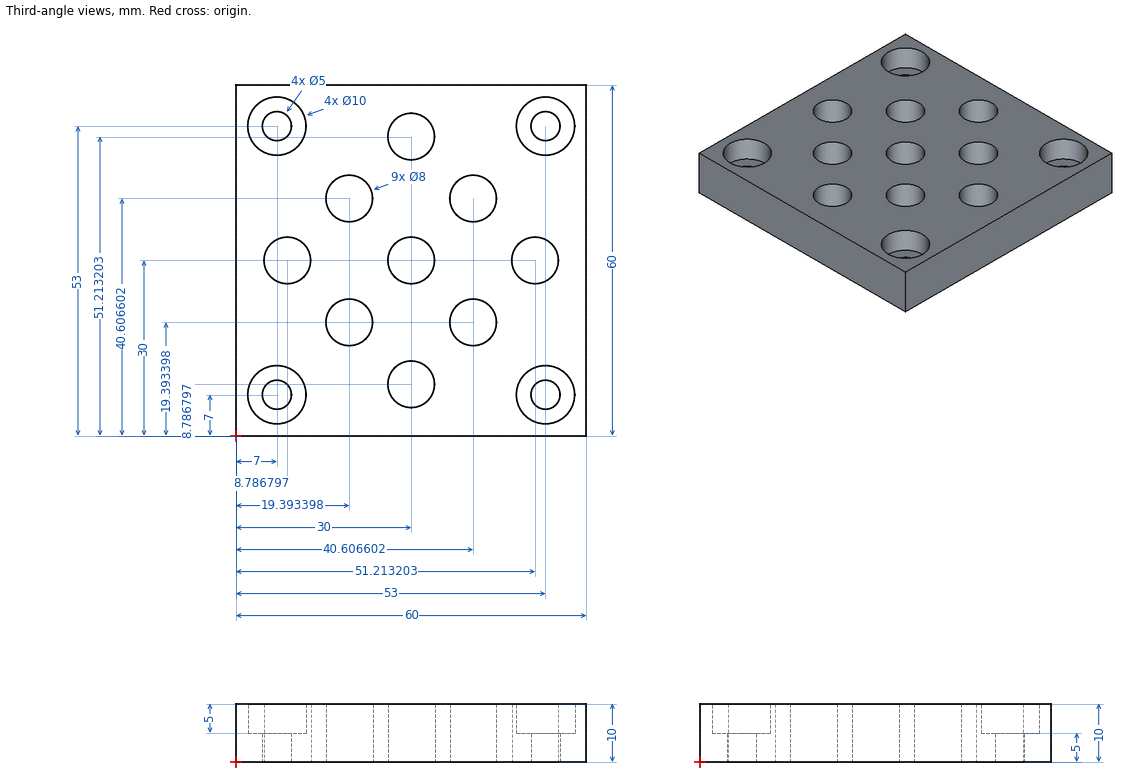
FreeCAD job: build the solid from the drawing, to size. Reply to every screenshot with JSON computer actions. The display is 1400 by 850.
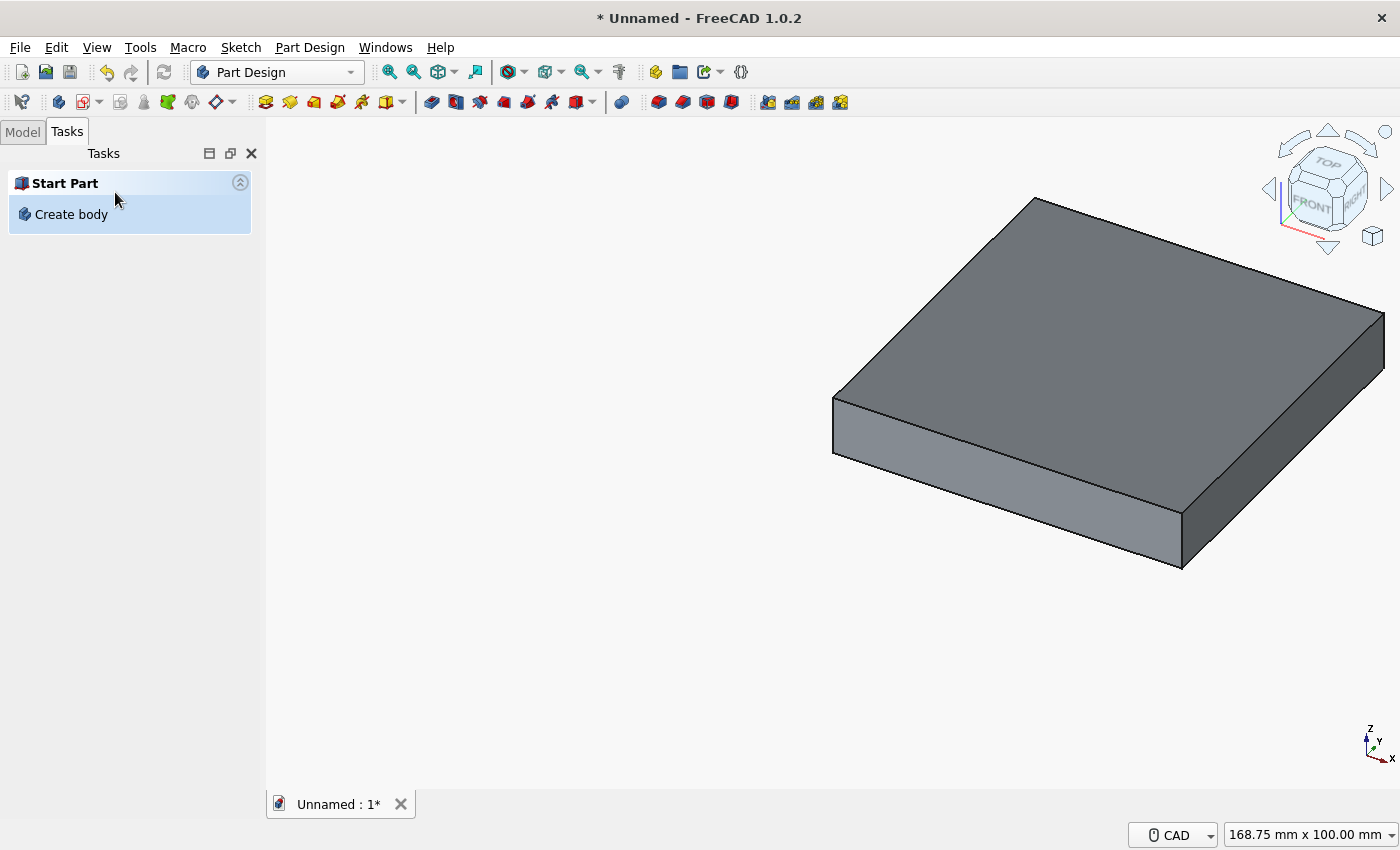
{"action": "left_click", "coordinate": [1108, 355]}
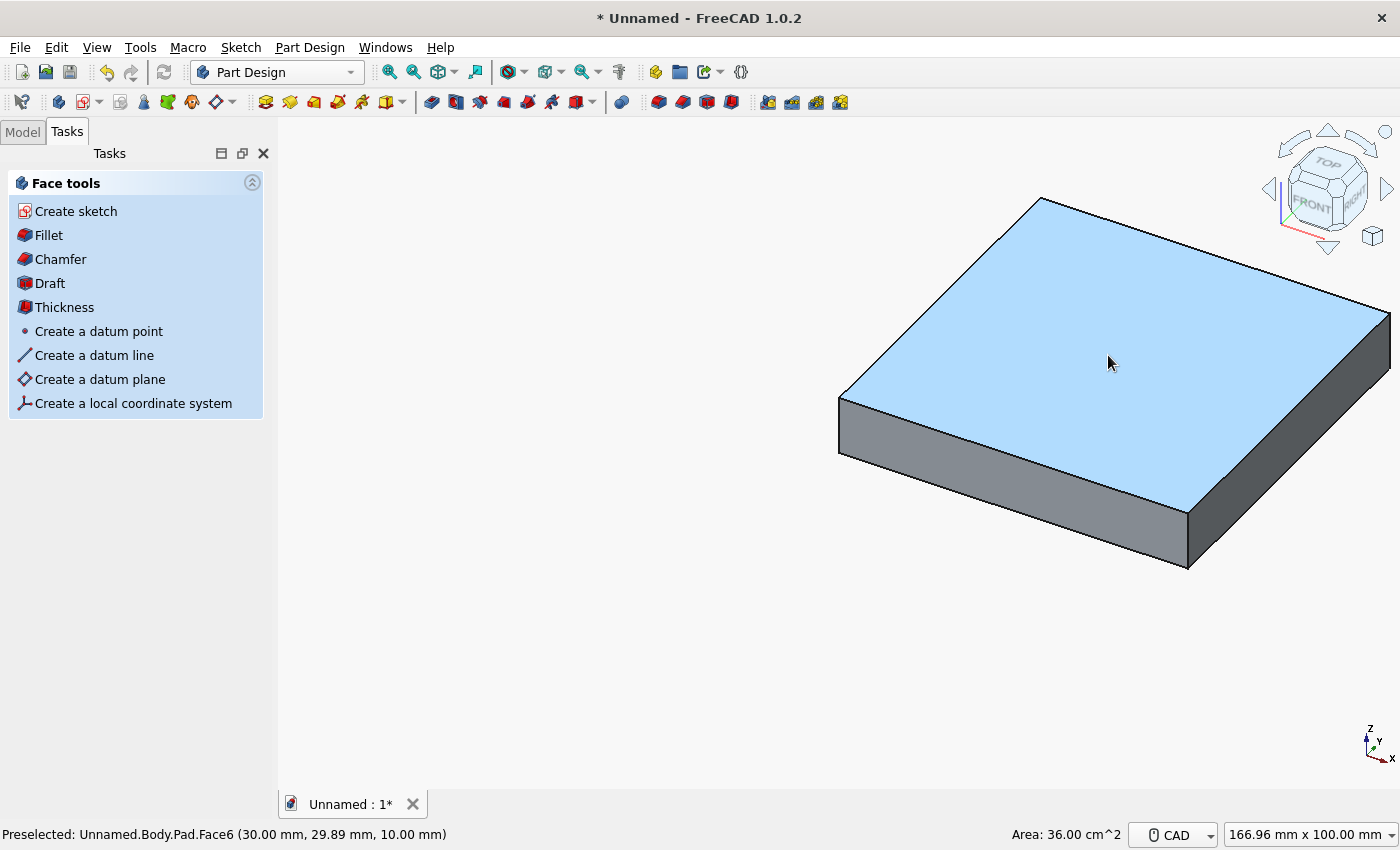
{"action": "left_click", "coordinate": [84, 102]}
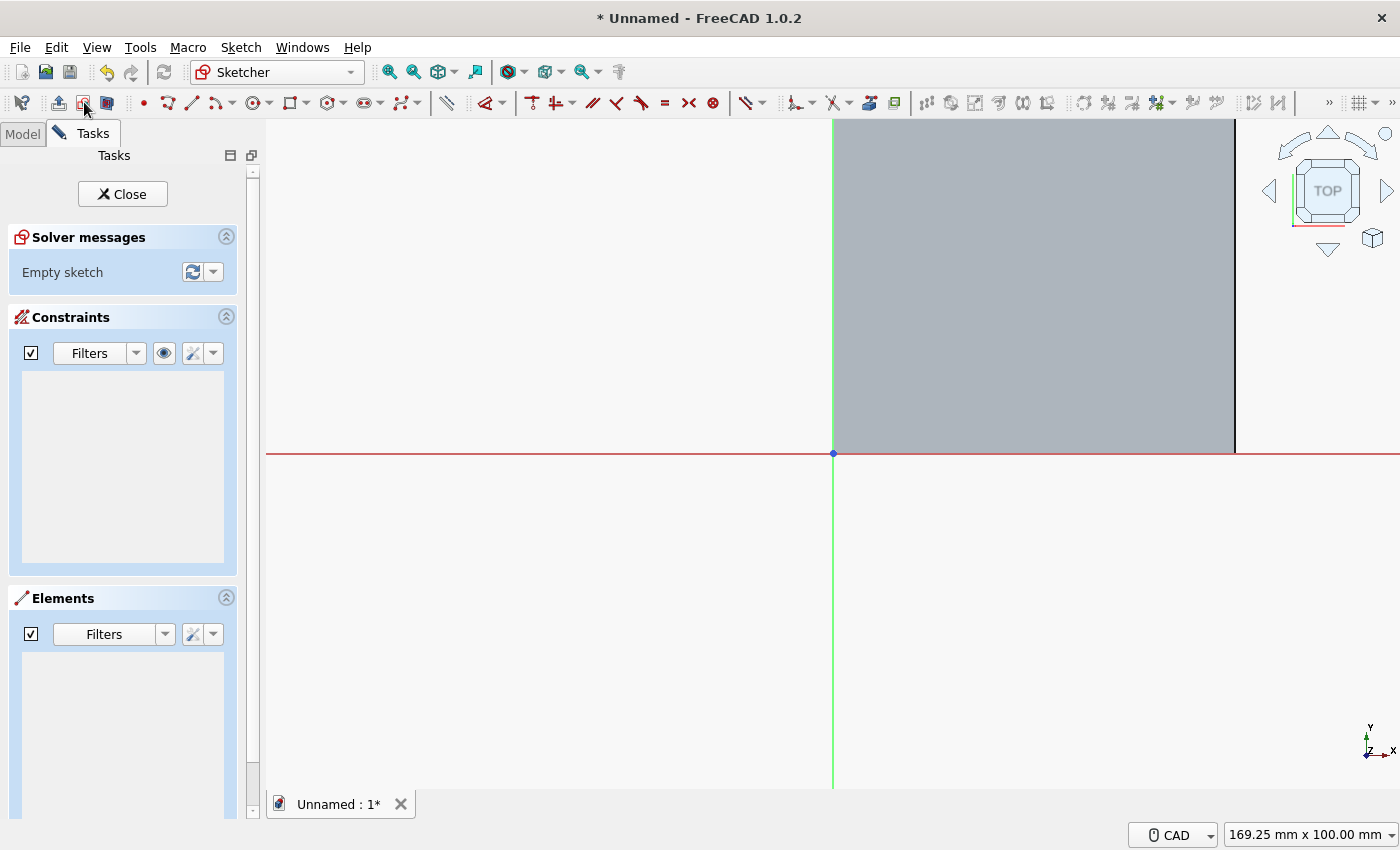
{"action": "scroll", "coordinate": [294, 761], "scroll_direction": "down", "scroll_amount": 1}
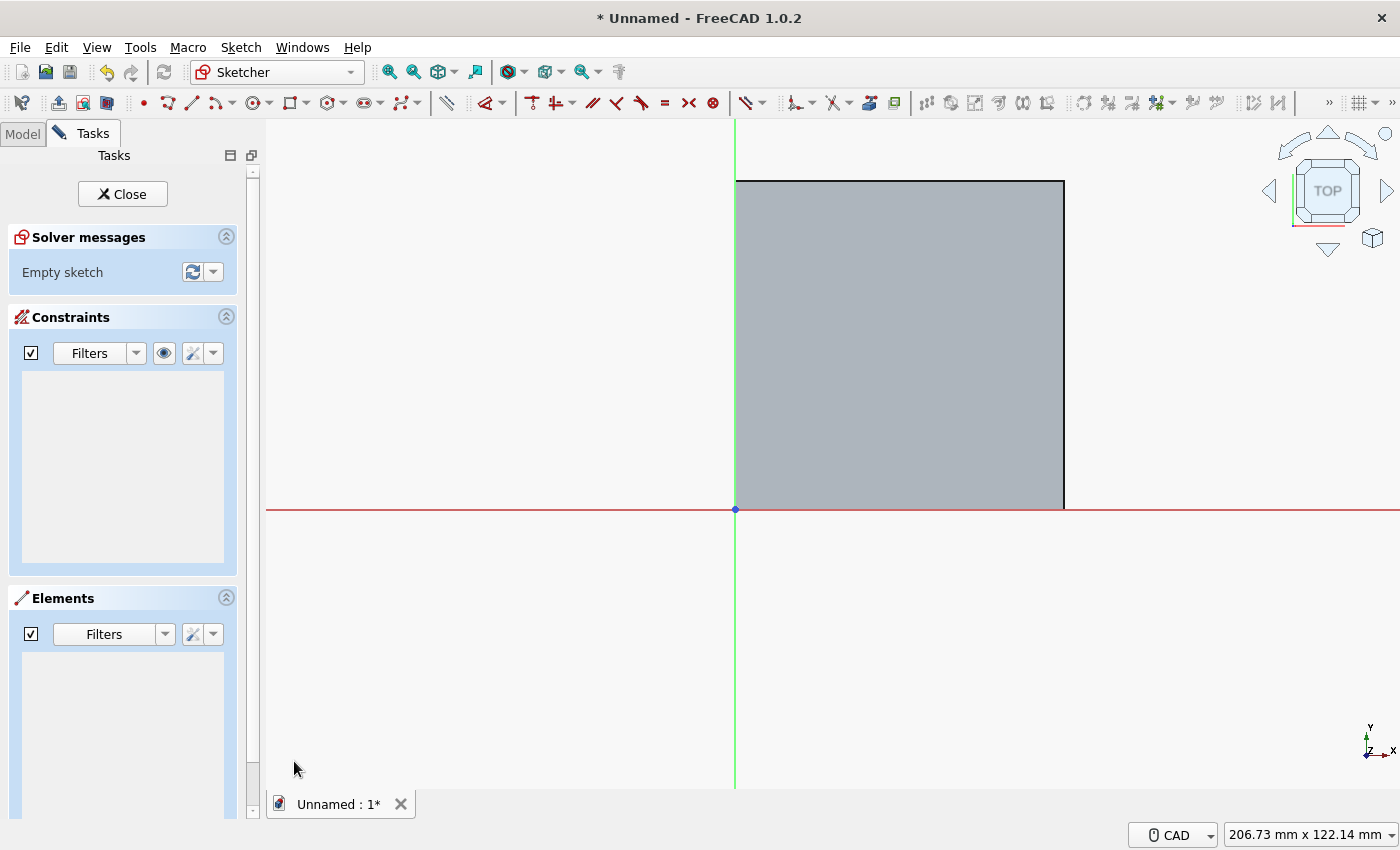
{"action": "scroll", "coordinate": [1158, 147], "scroll_direction": "up", "scroll_amount": 2}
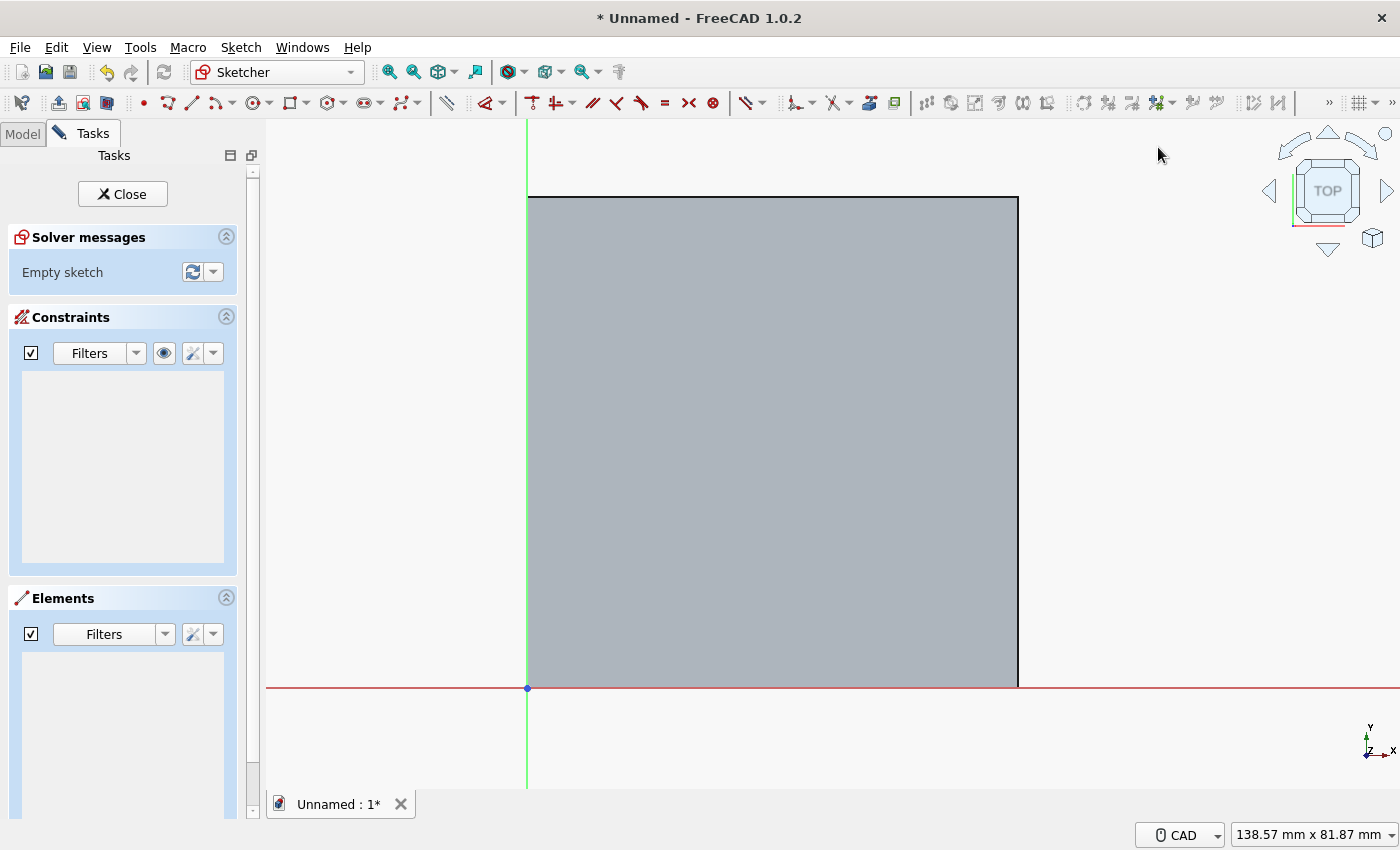
{"action": "left_click", "coordinate": [254, 104]}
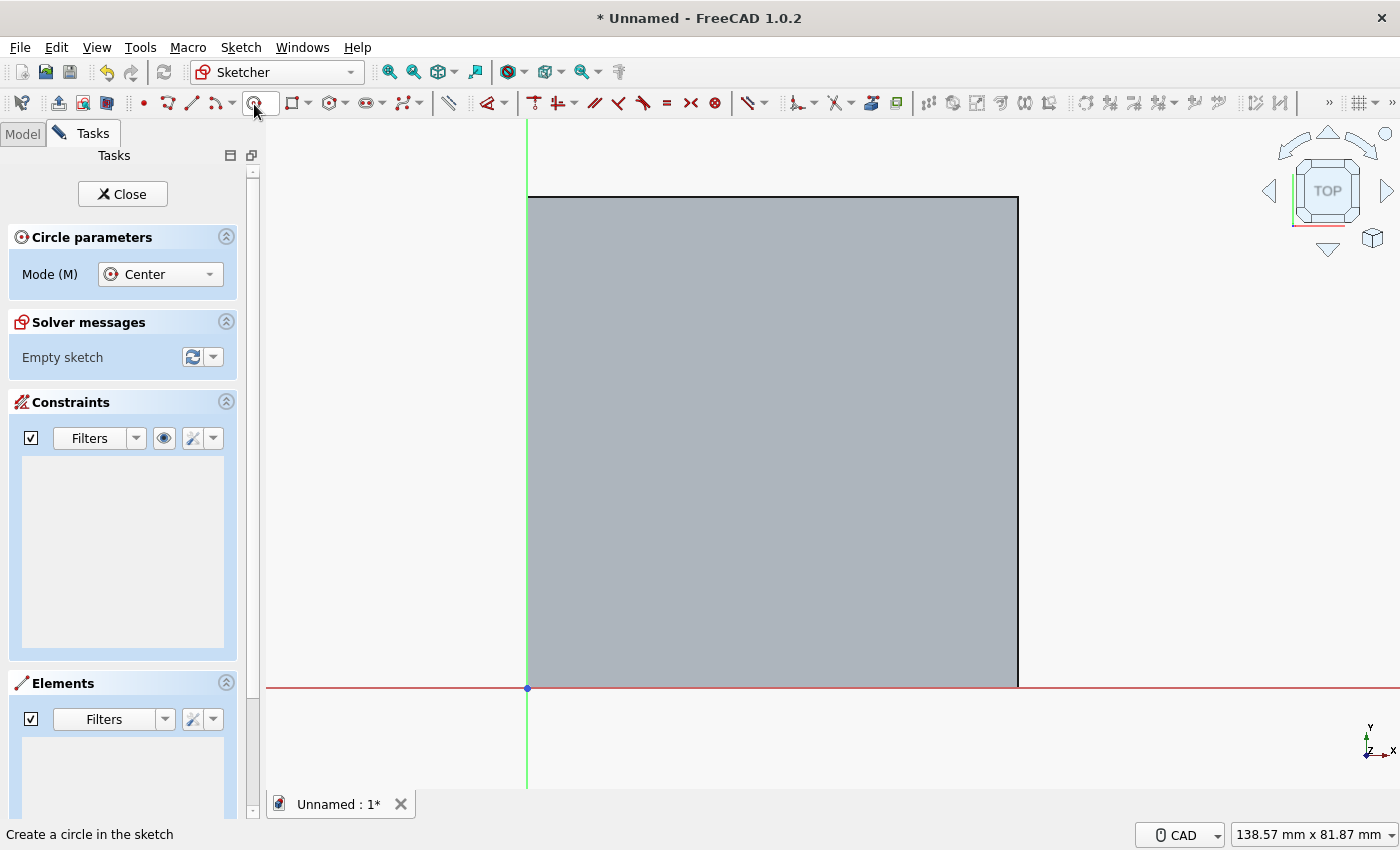
{"action": "left_click", "coordinate": [584, 255]}
{"action": "left_click", "coordinate": [613, 226]}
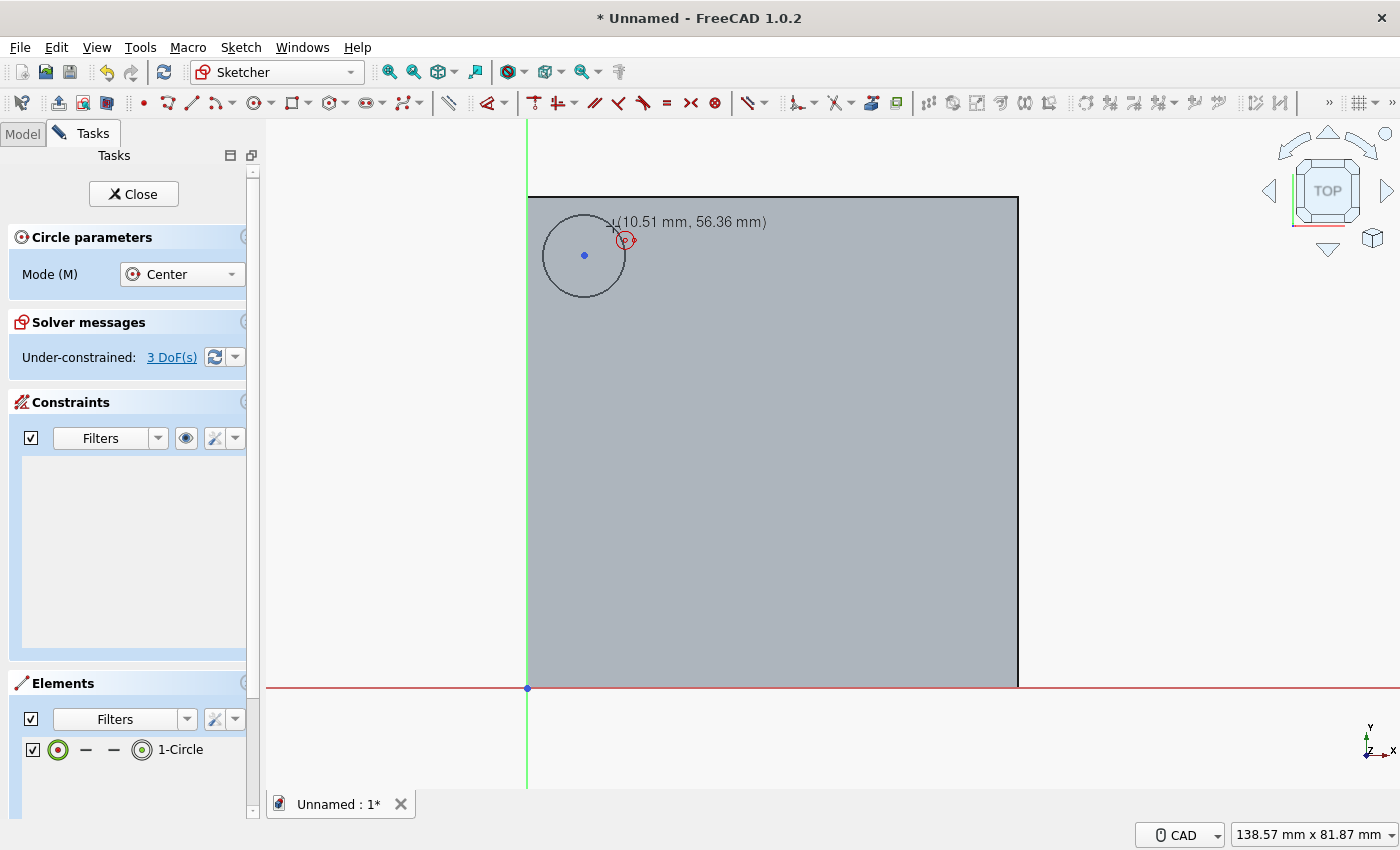
{"action": "left_click", "coordinate": [961, 255]}
{"action": "left_click", "coordinate": [990, 226]}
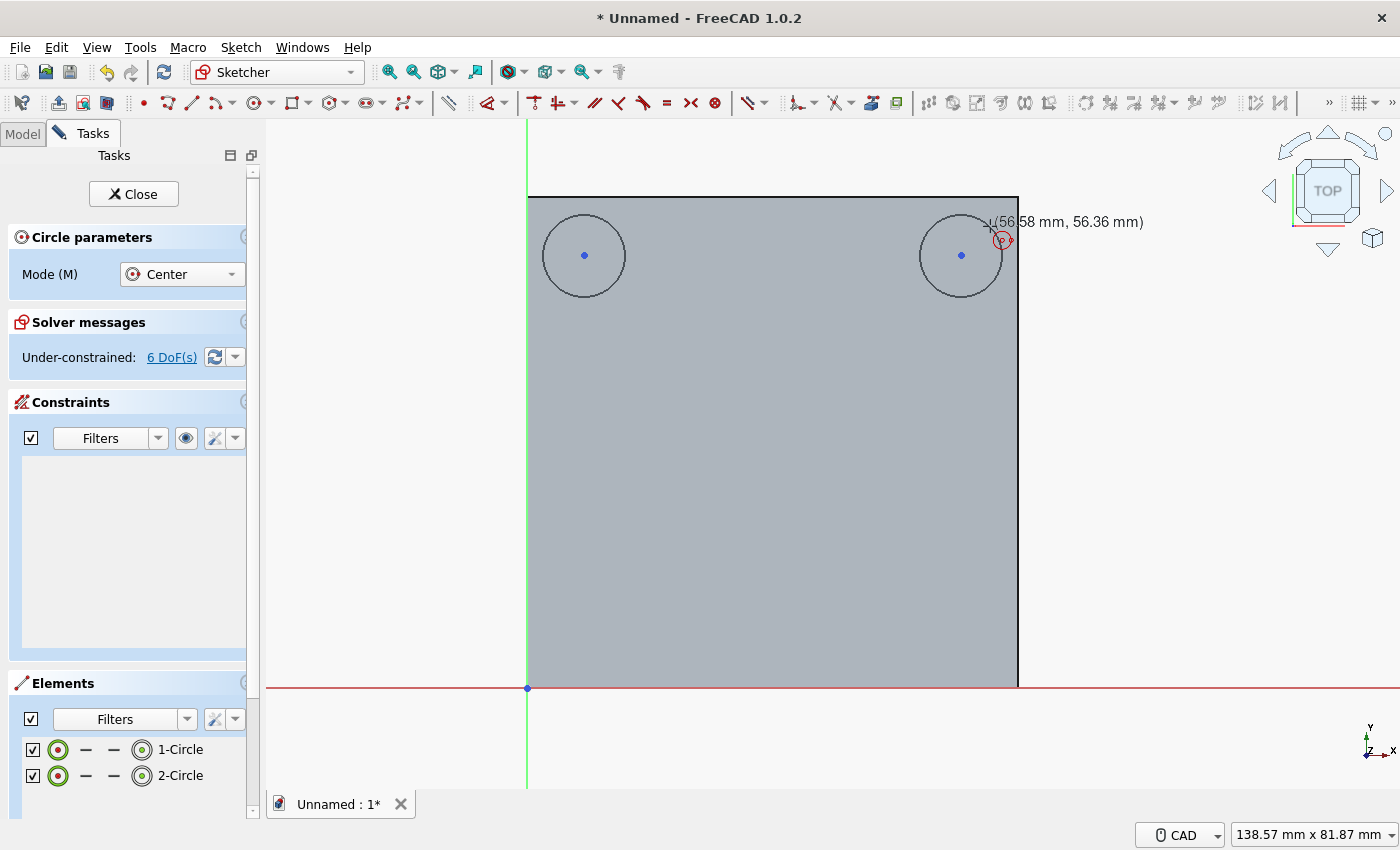
{"action": "left_click", "coordinate": [584, 631]}
{"action": "left_click", "coordinate": [613, 602]}